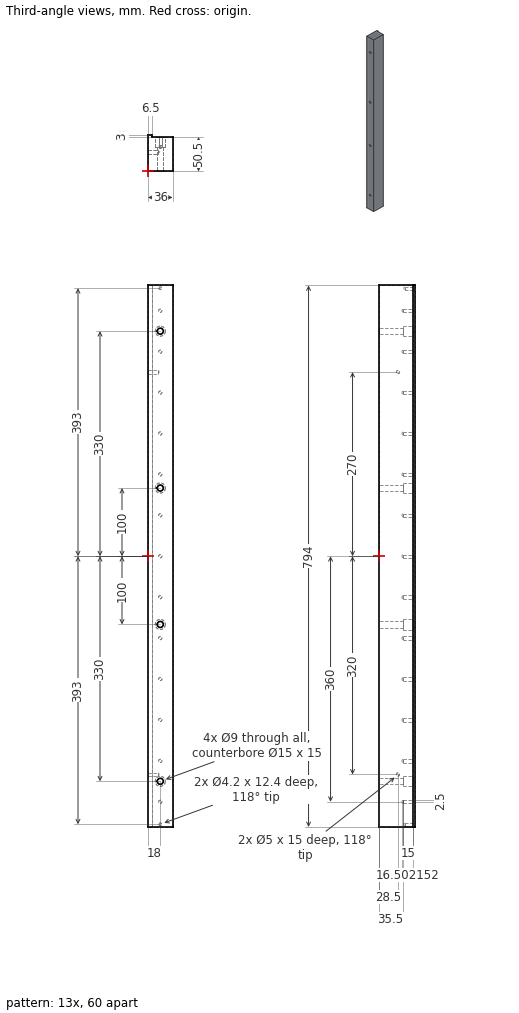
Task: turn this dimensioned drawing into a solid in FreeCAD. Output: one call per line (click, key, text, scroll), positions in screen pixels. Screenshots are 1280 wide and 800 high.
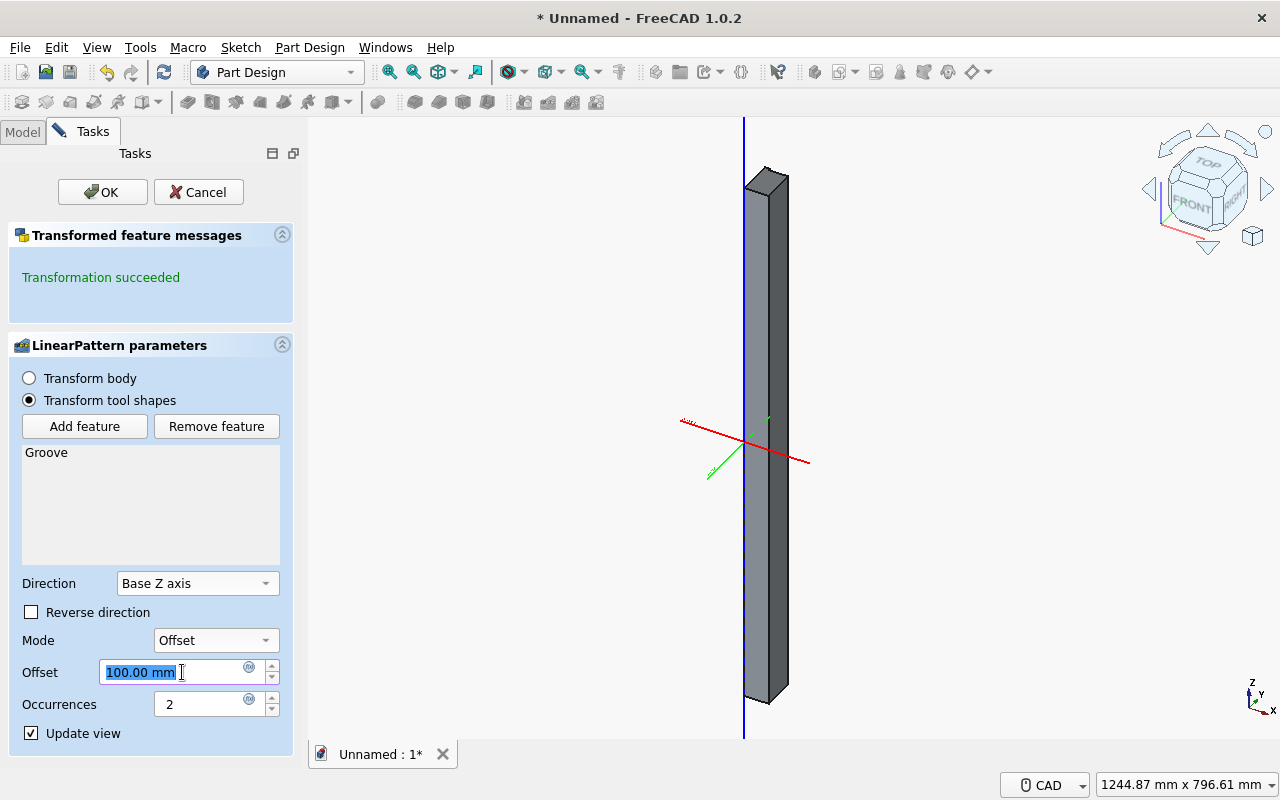
text(60)
key(Tab)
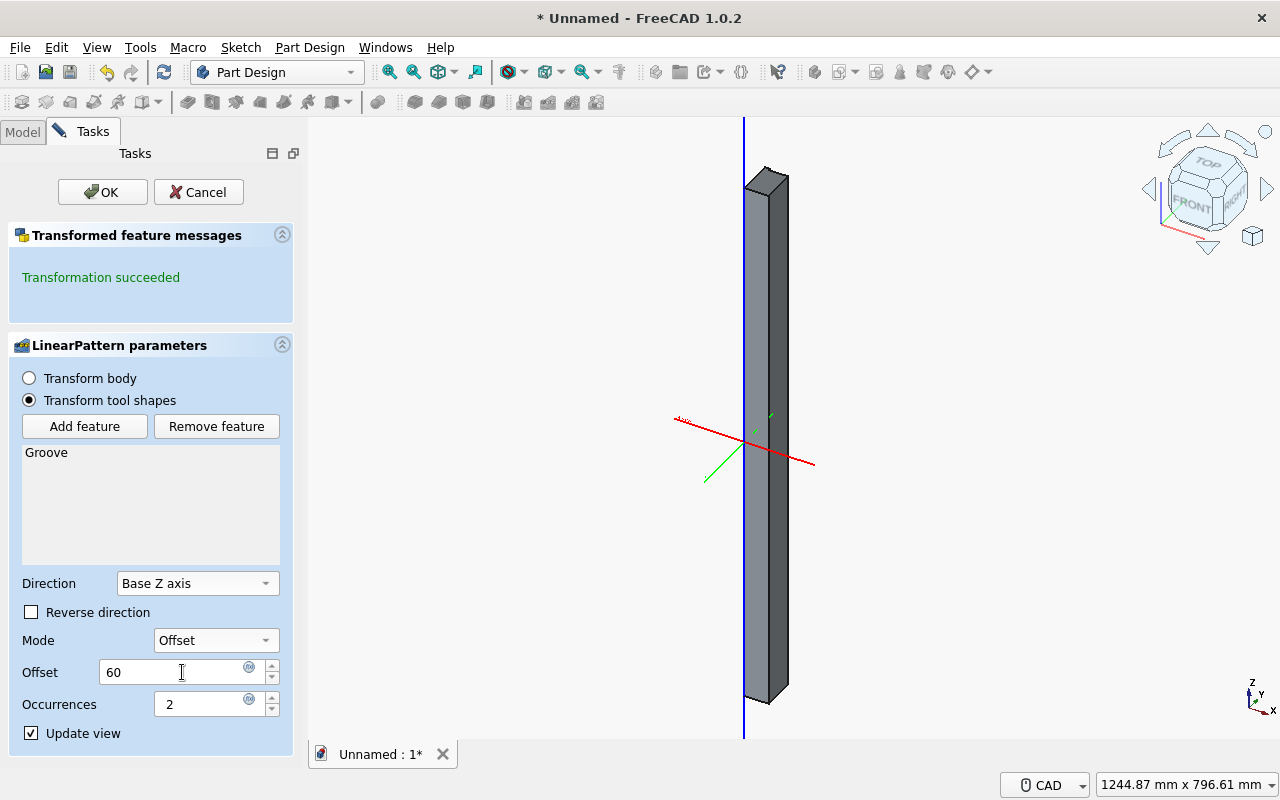
triple_click(209, 704)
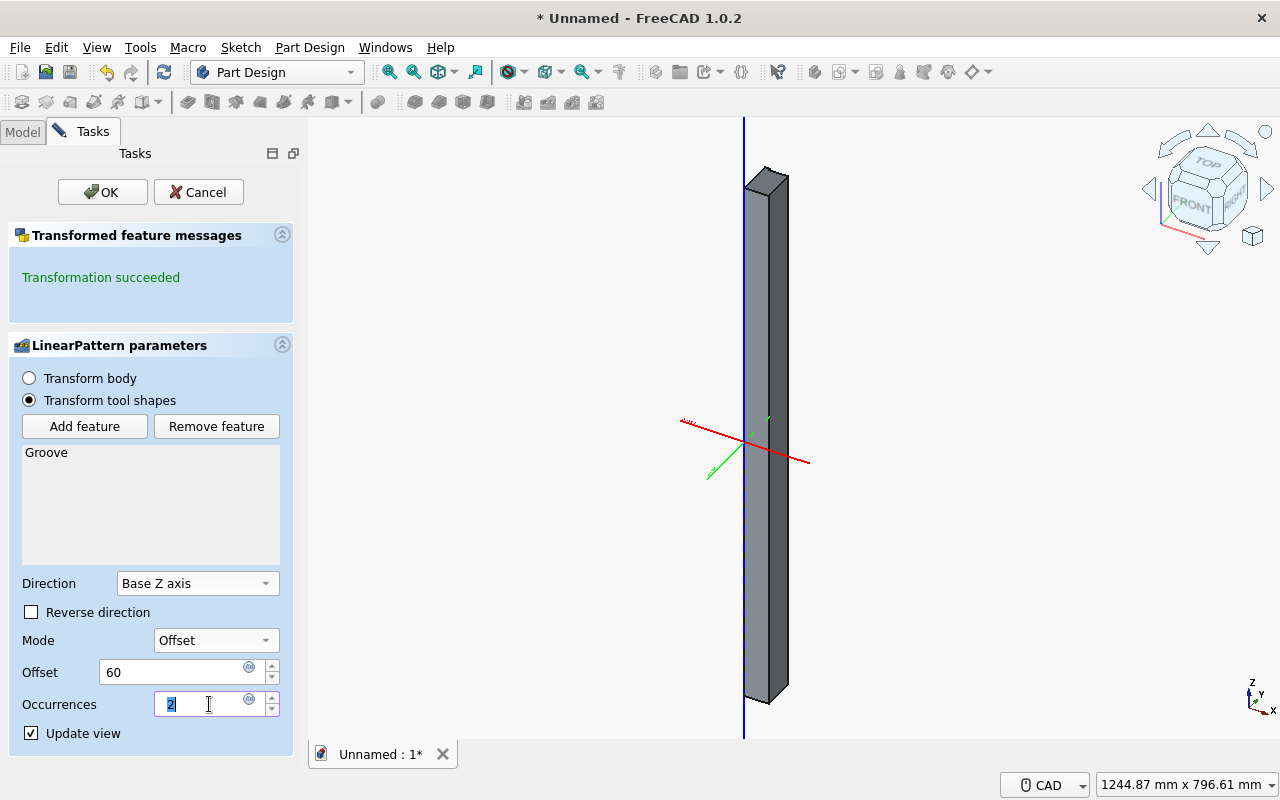
text(13)
key(Tab)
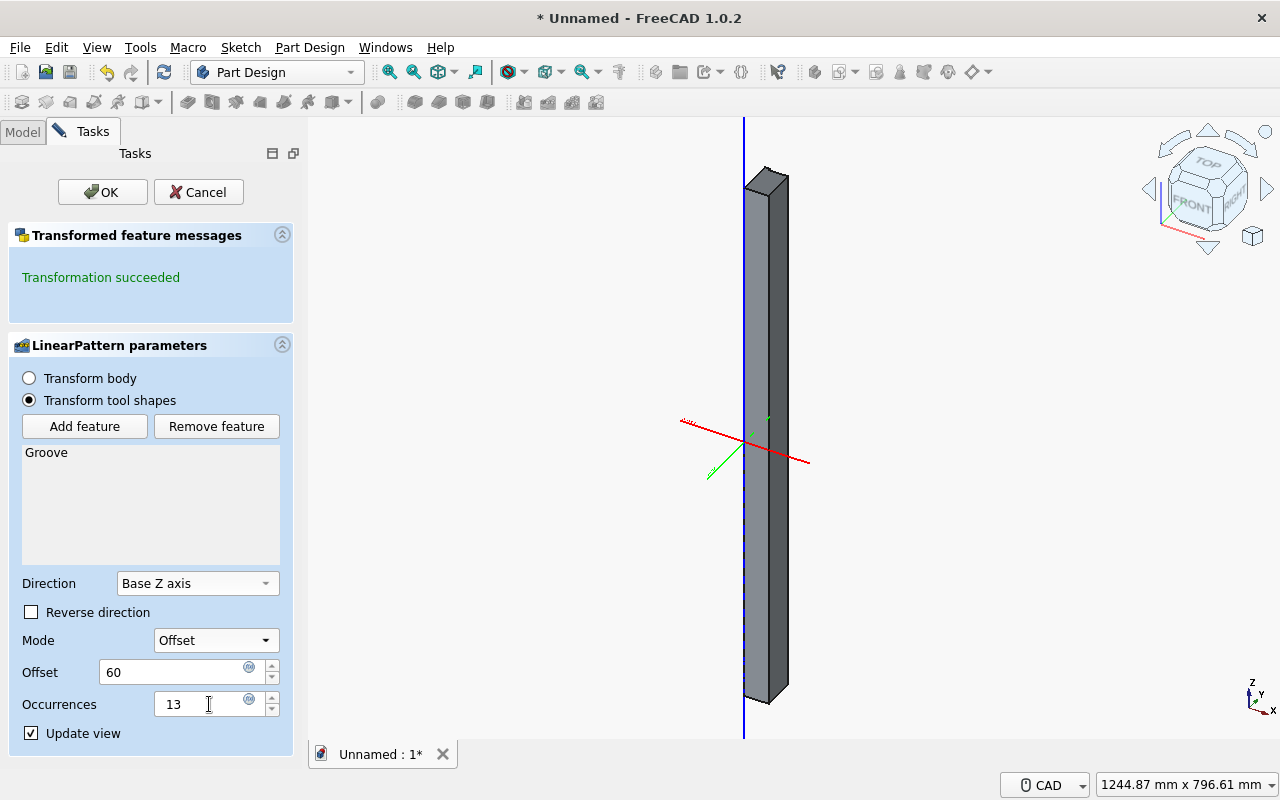
click(103, 192)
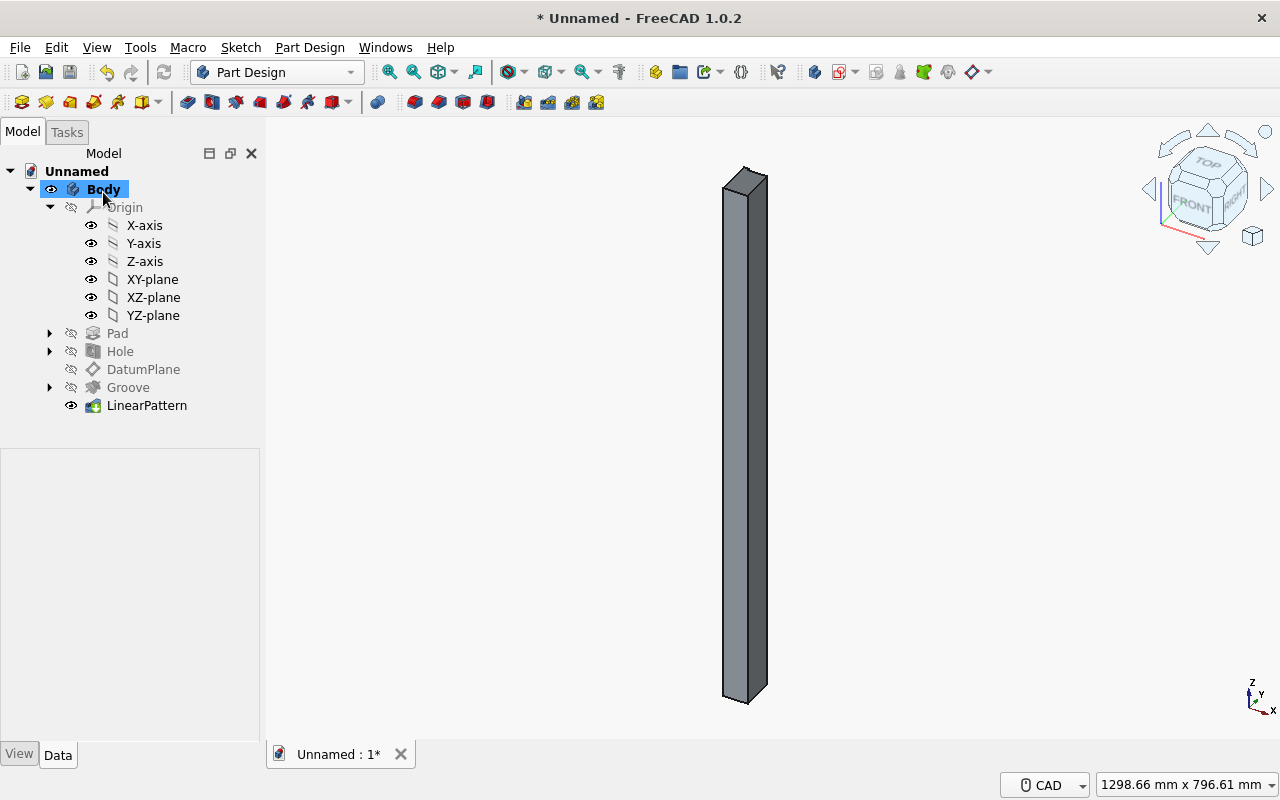
key(4)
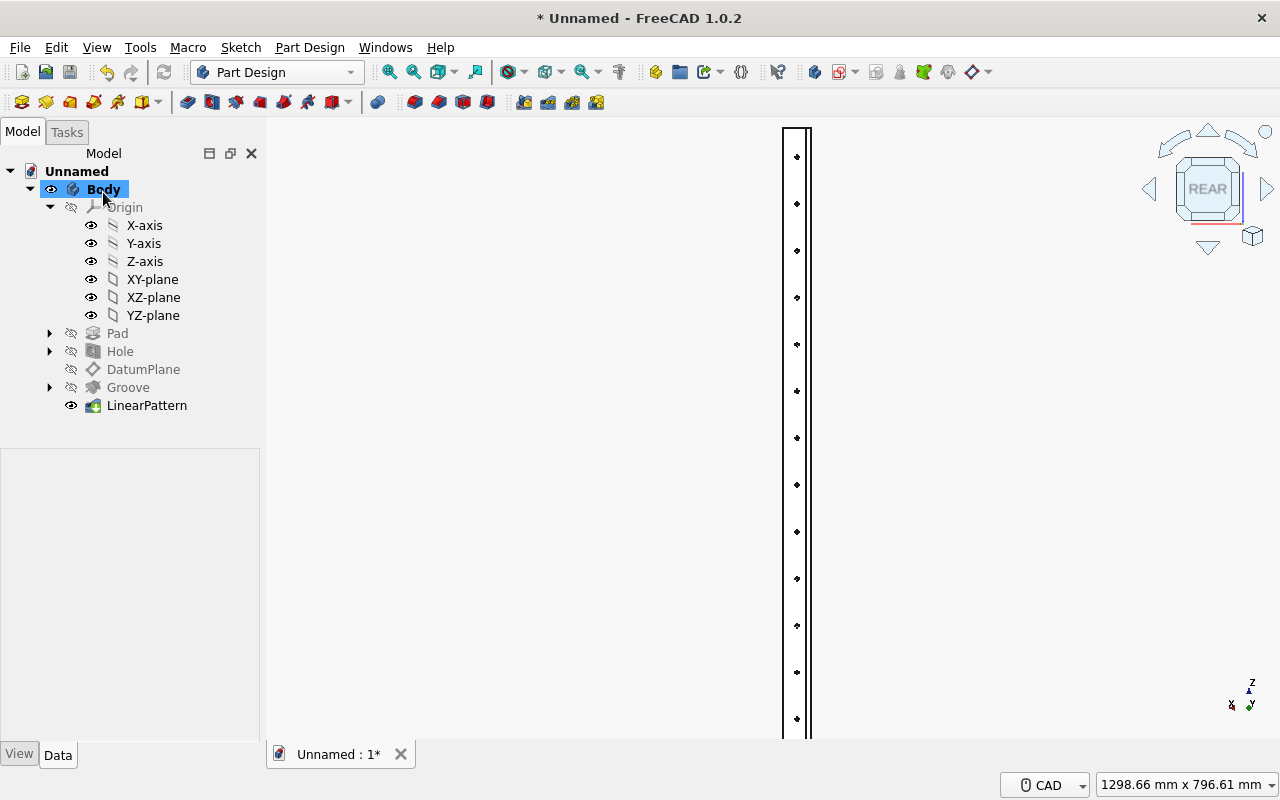
click(390, 72)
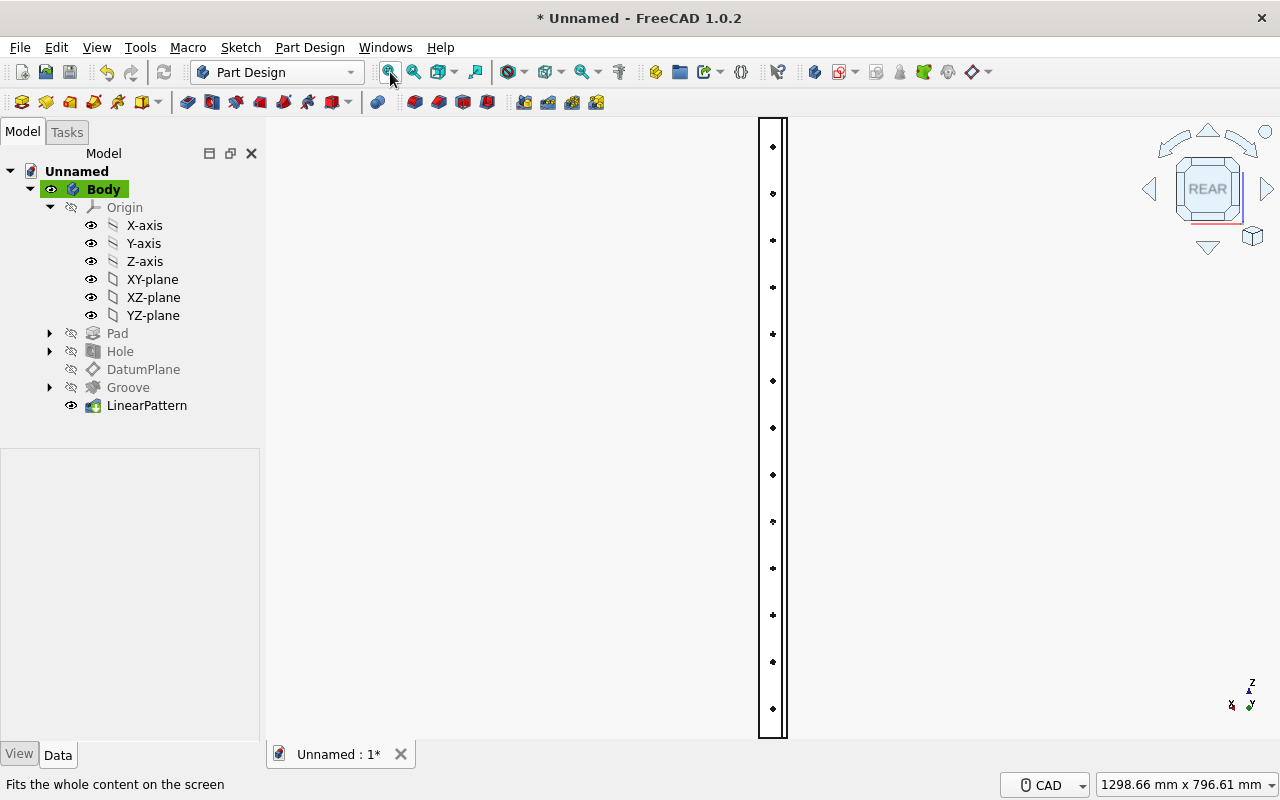
click(770, 161)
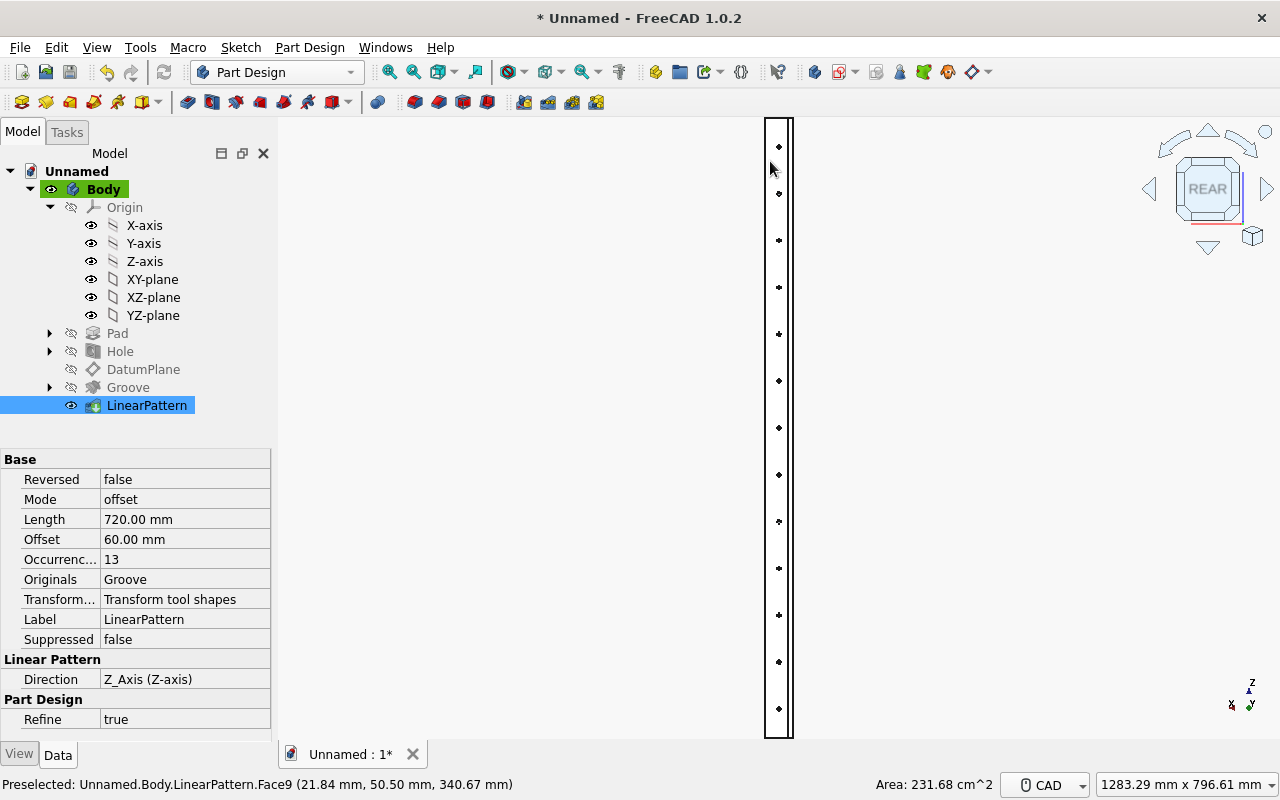
click(840, 72)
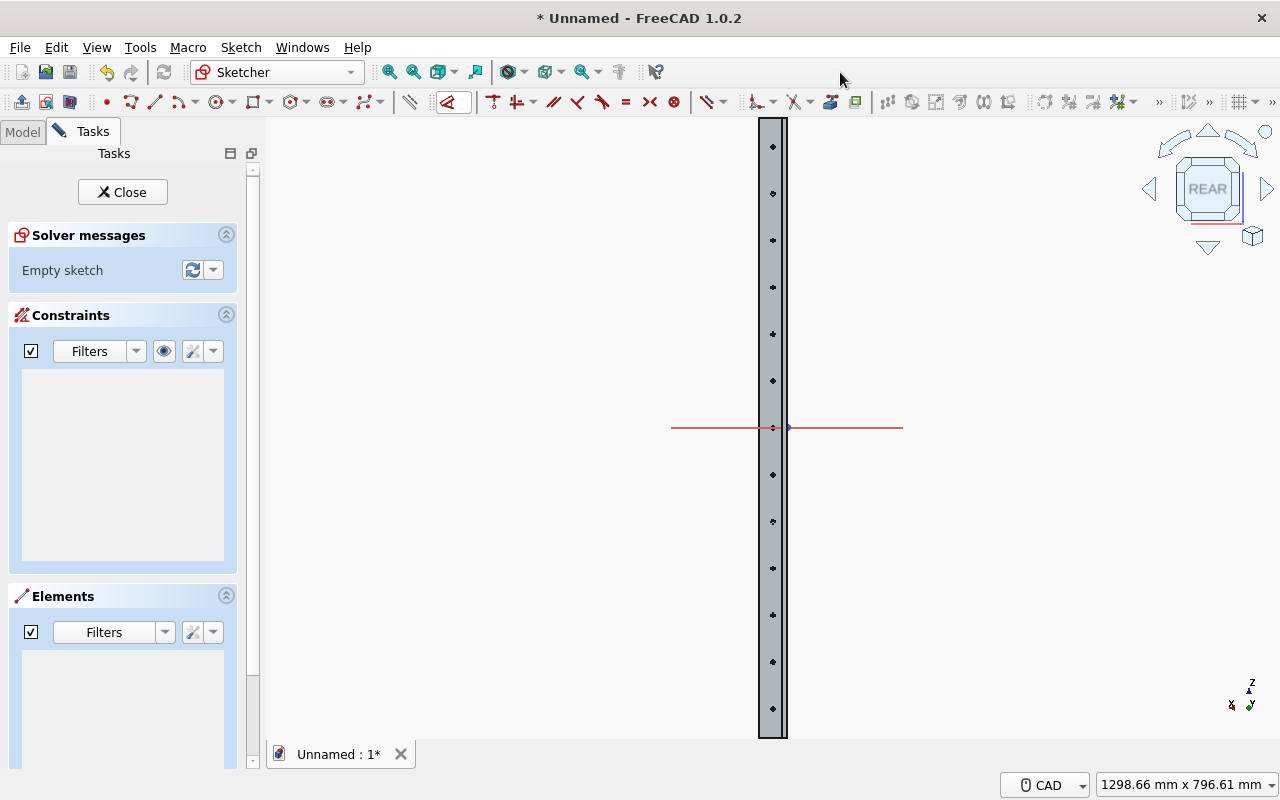
click(70, 102)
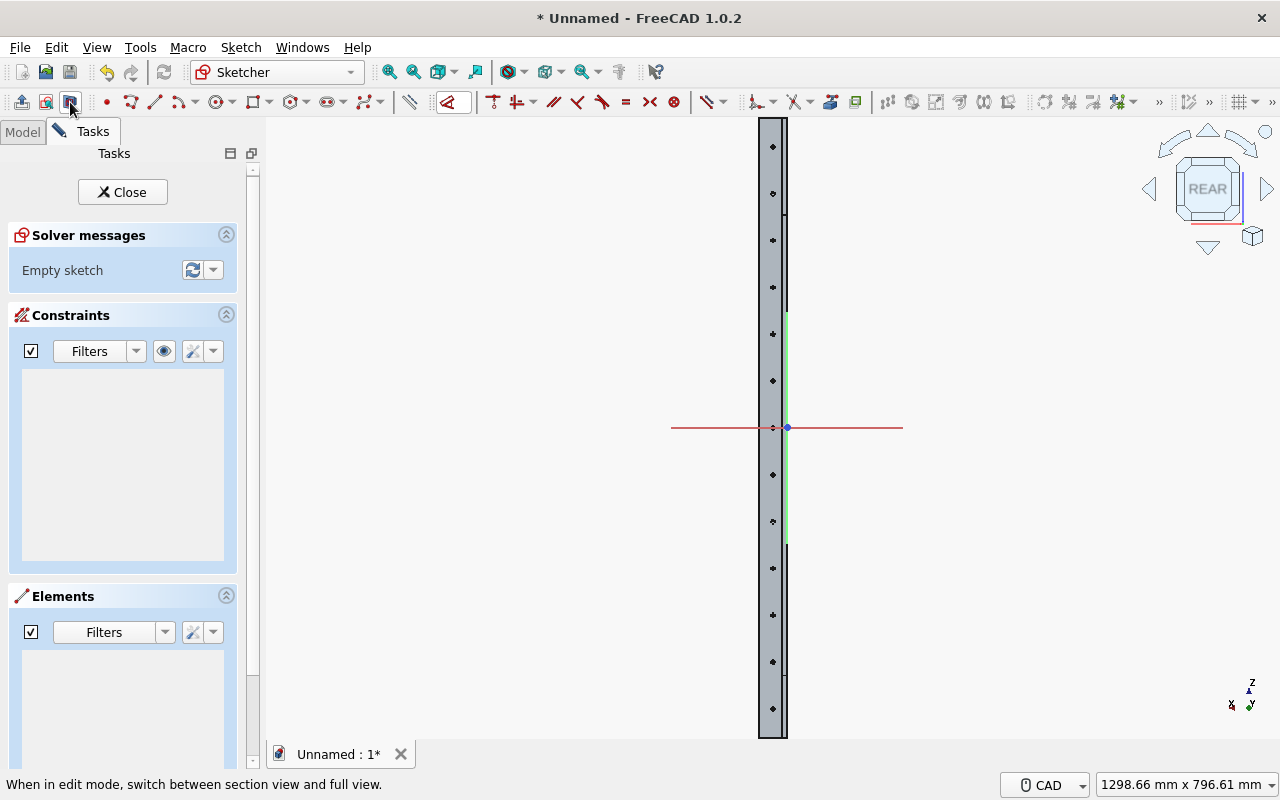
scroll(371, 428, down, 1)